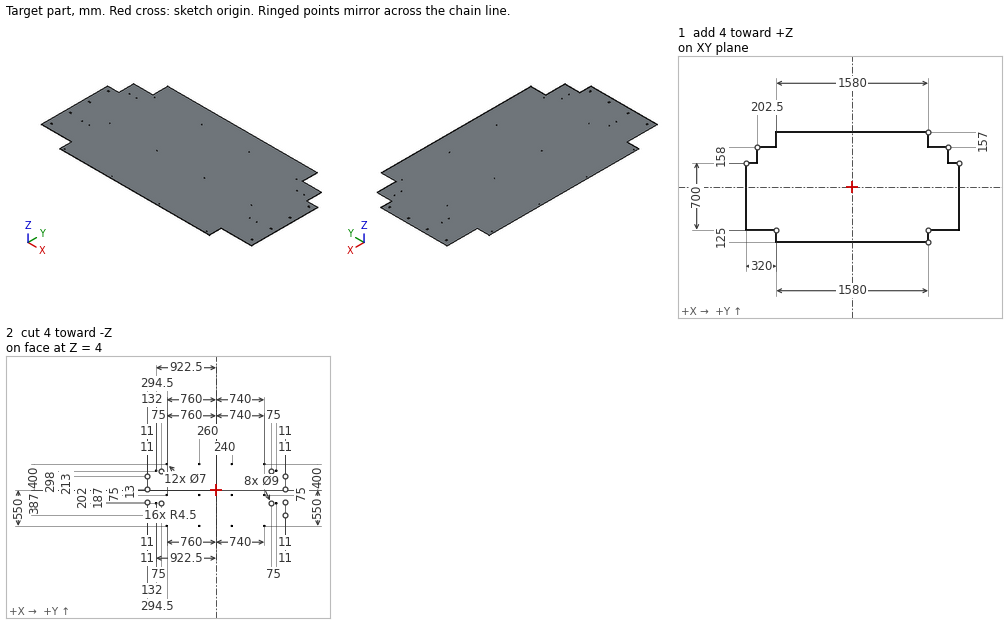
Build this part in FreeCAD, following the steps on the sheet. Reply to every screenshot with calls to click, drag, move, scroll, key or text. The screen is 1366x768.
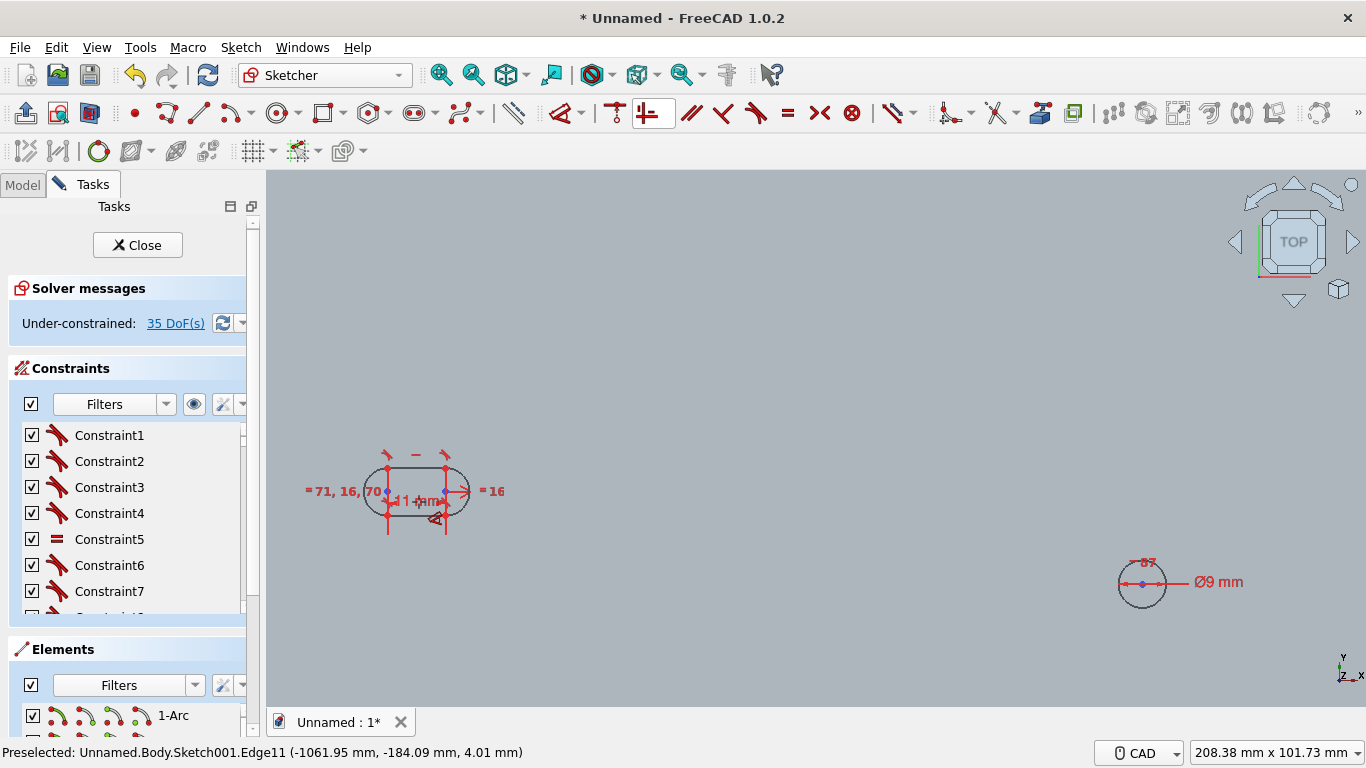
scroll(406, 474, down, 14)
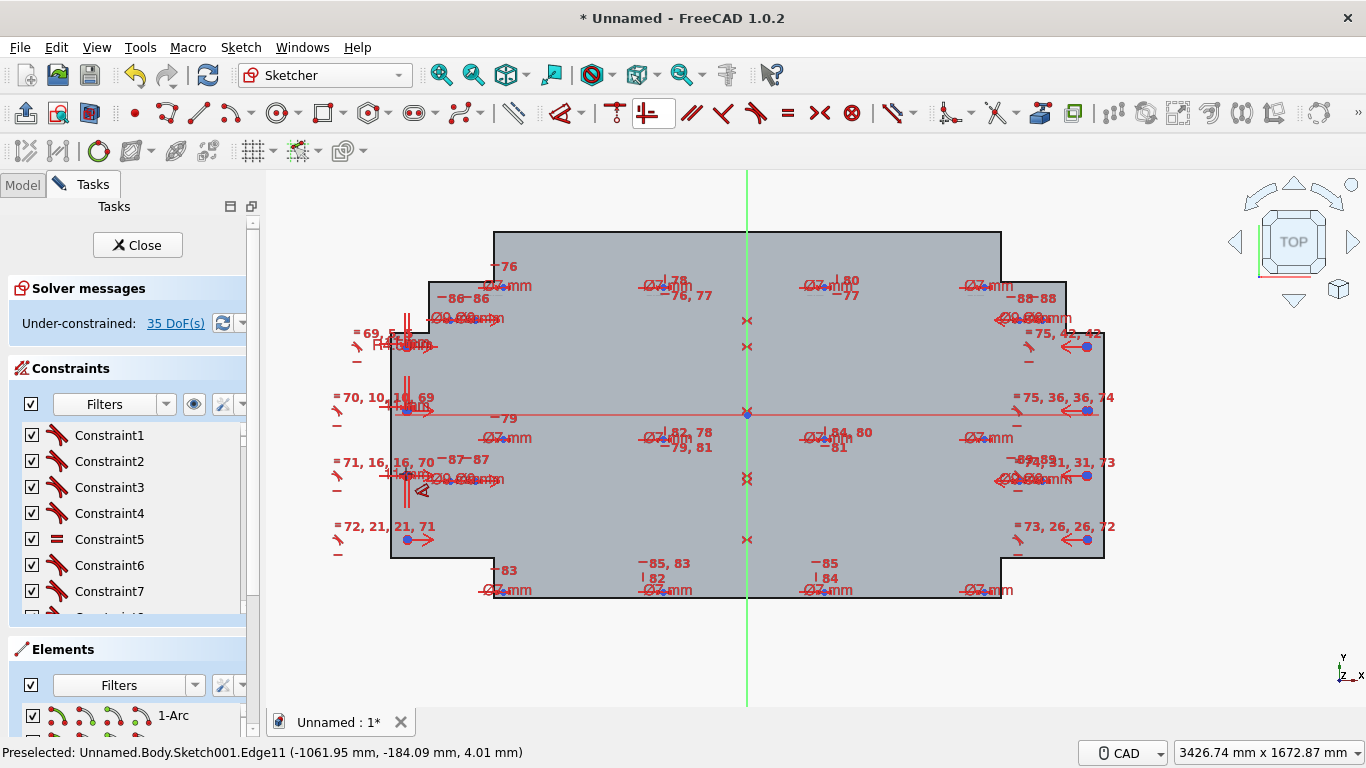
scroll(407, 538, up, 14)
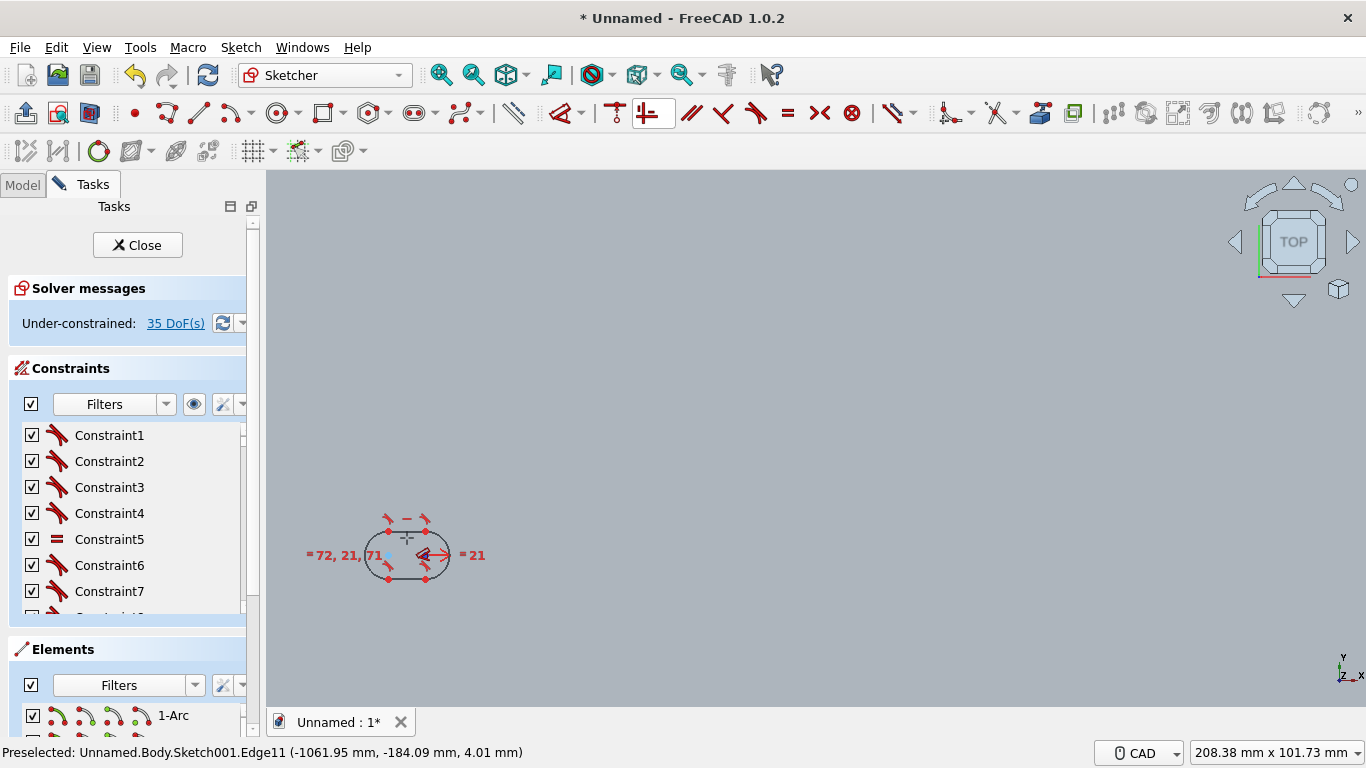
click(400, 532)
click(407, 566)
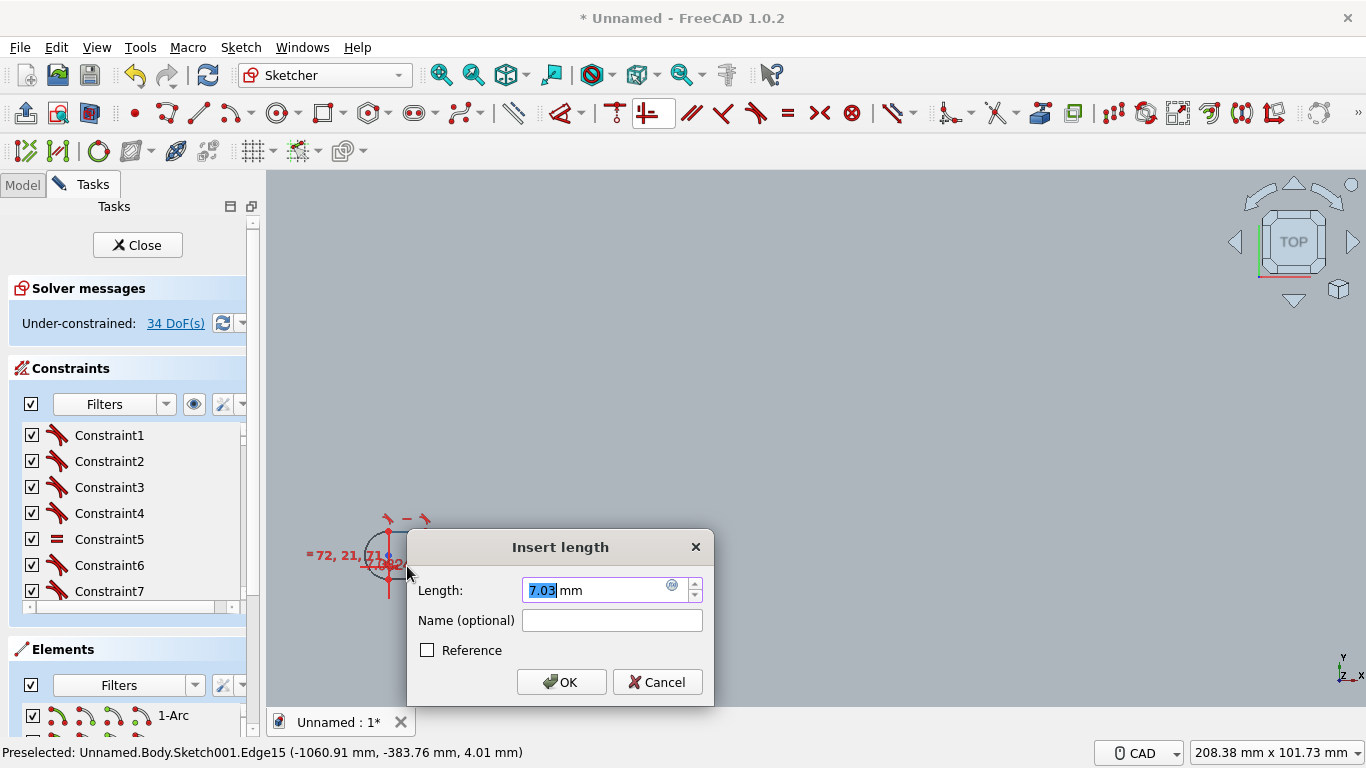
text(11)
key(Return)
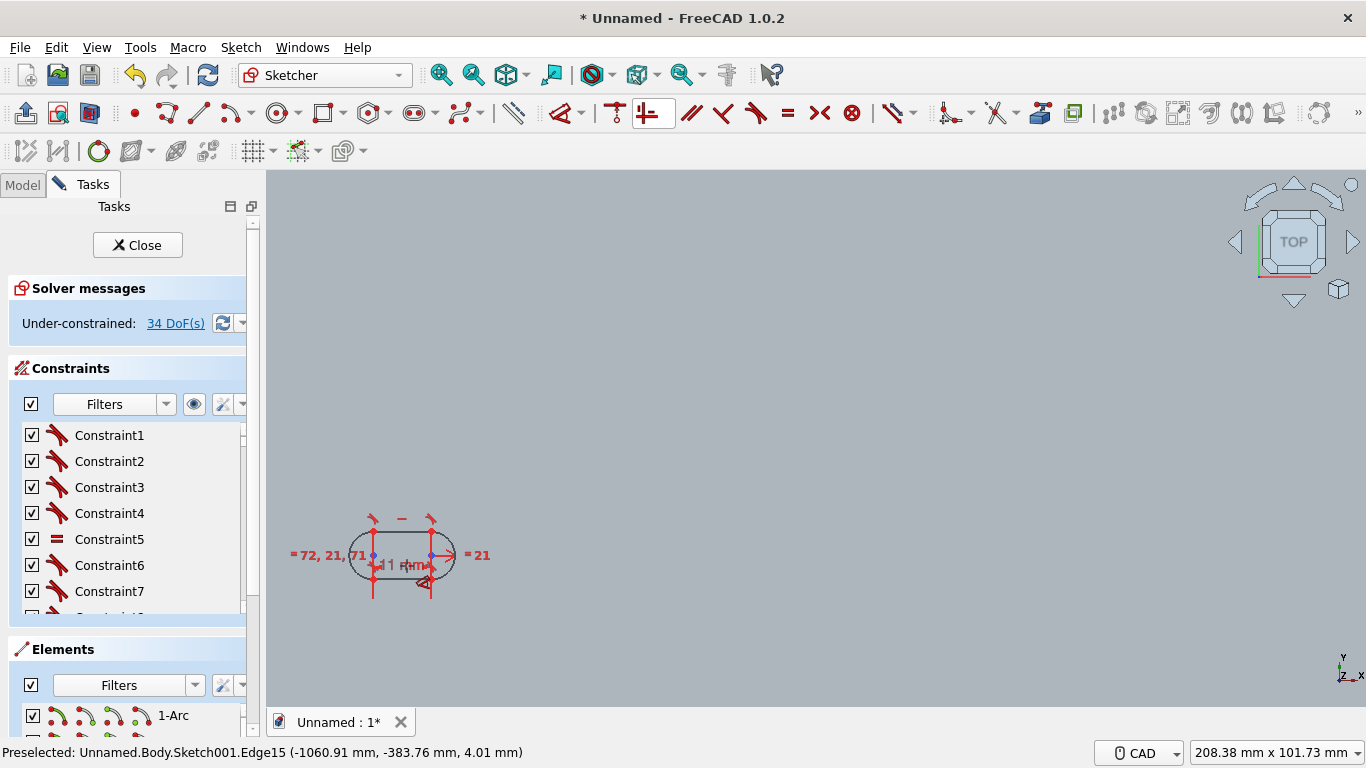
scroll(407, 538, down, 14)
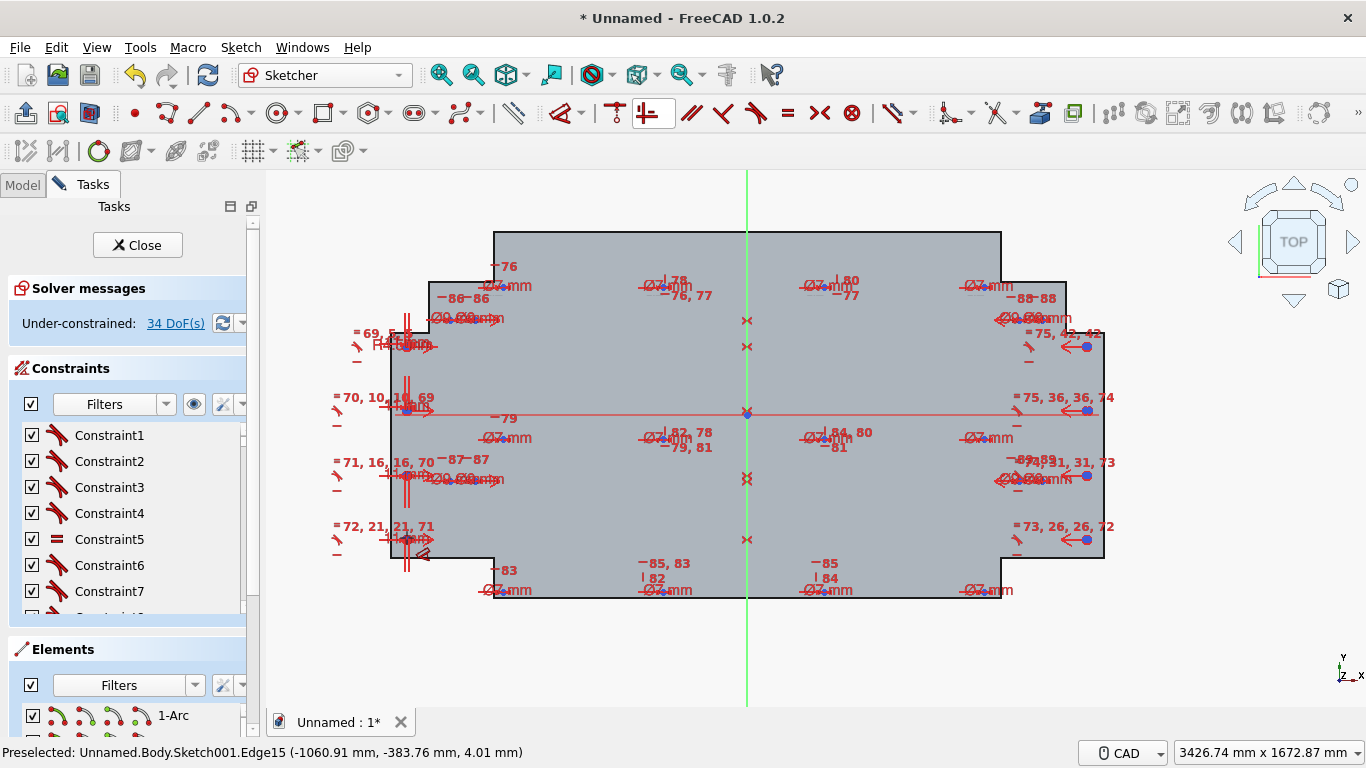
scroll(1087, 538, up, 14)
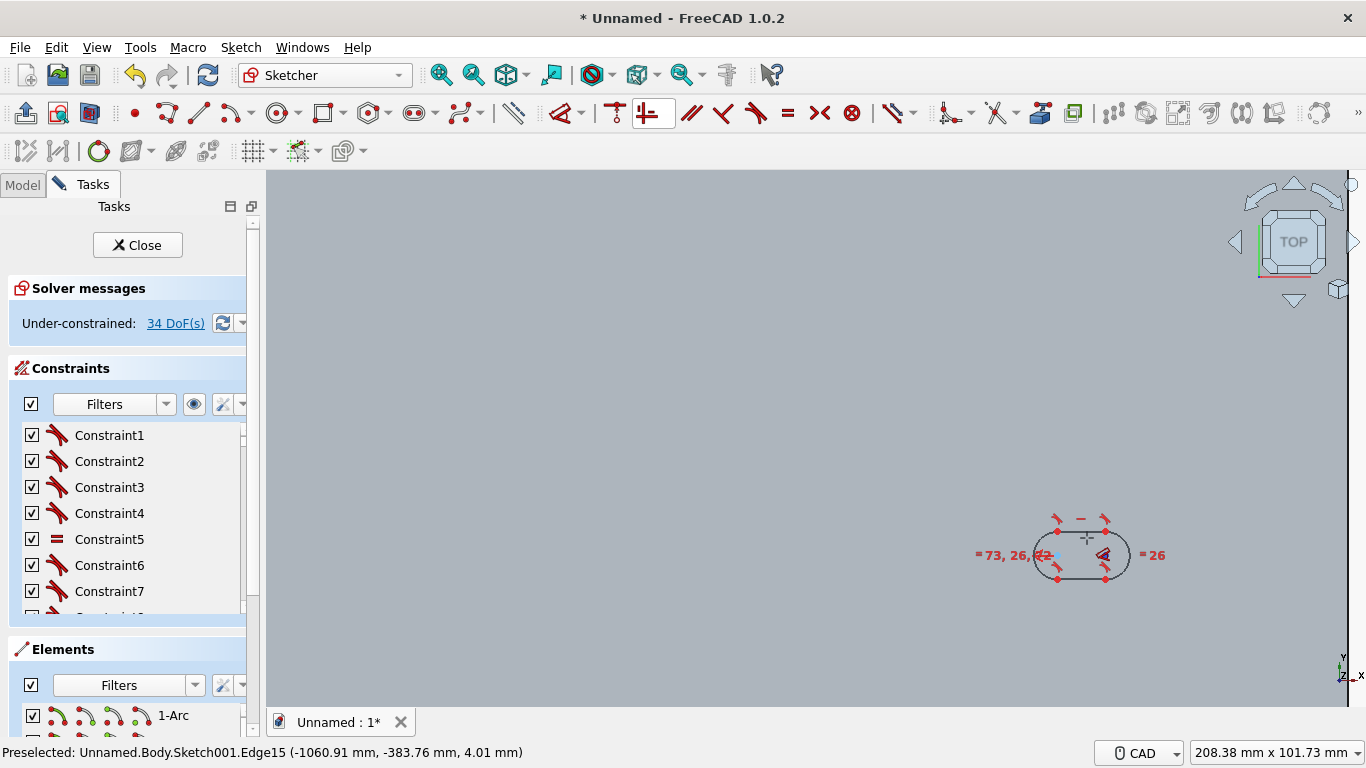
click(1072, 532)
click(1082, 566)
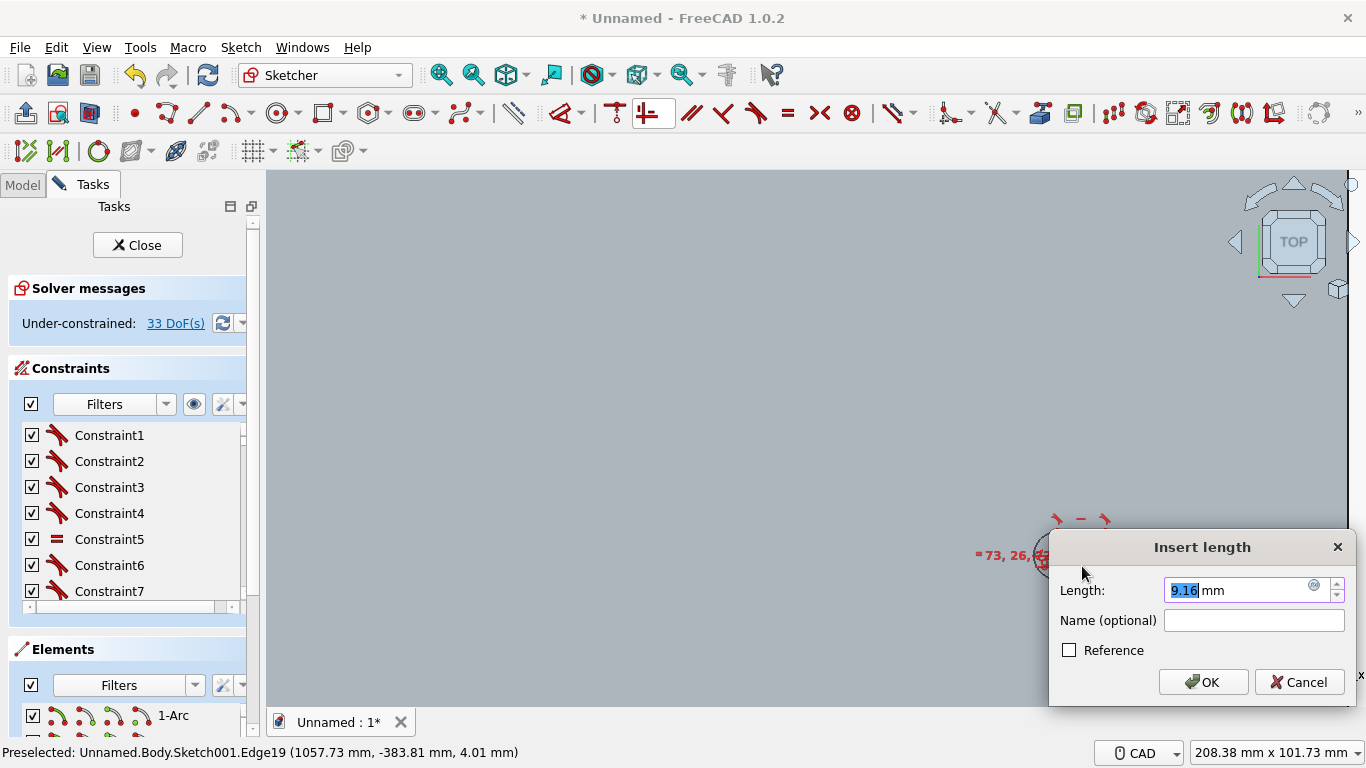
text(11)
key(Return)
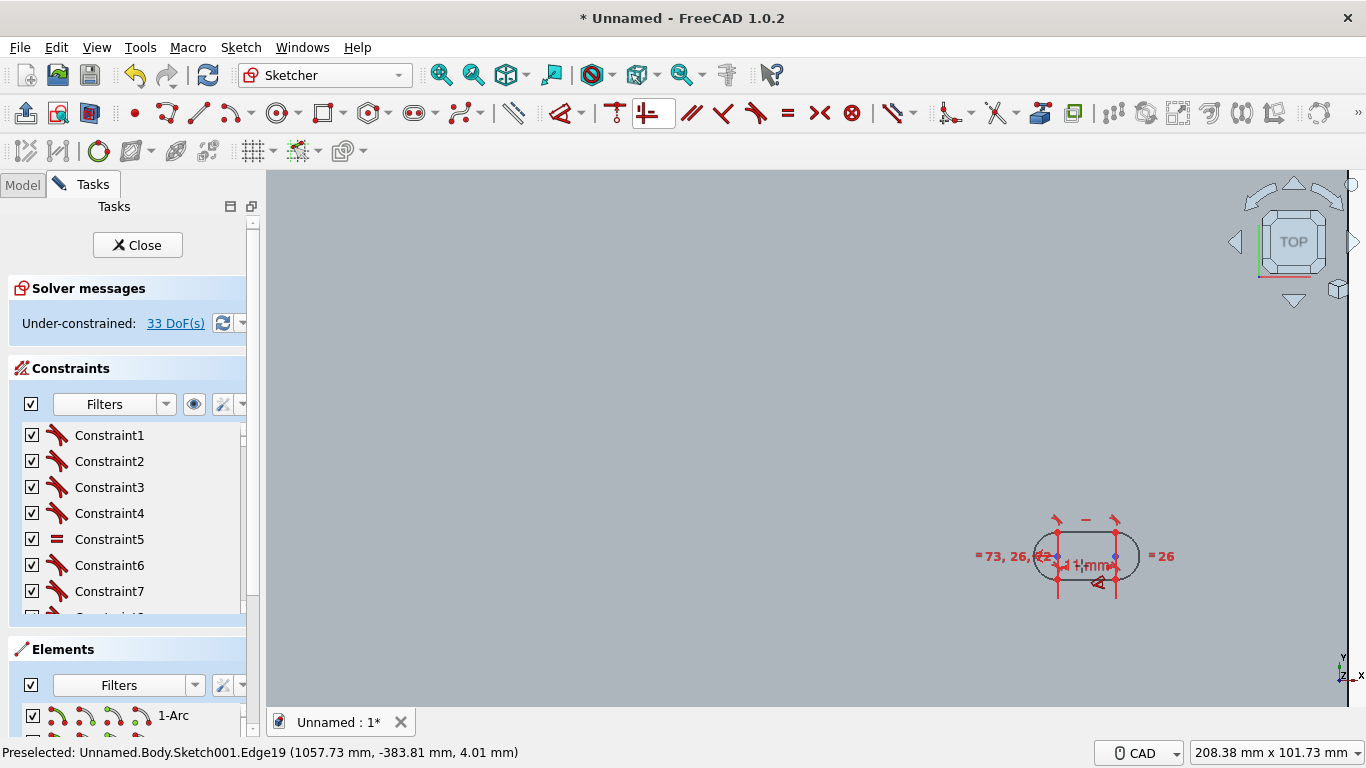
scroll(1088, 538, down, 14)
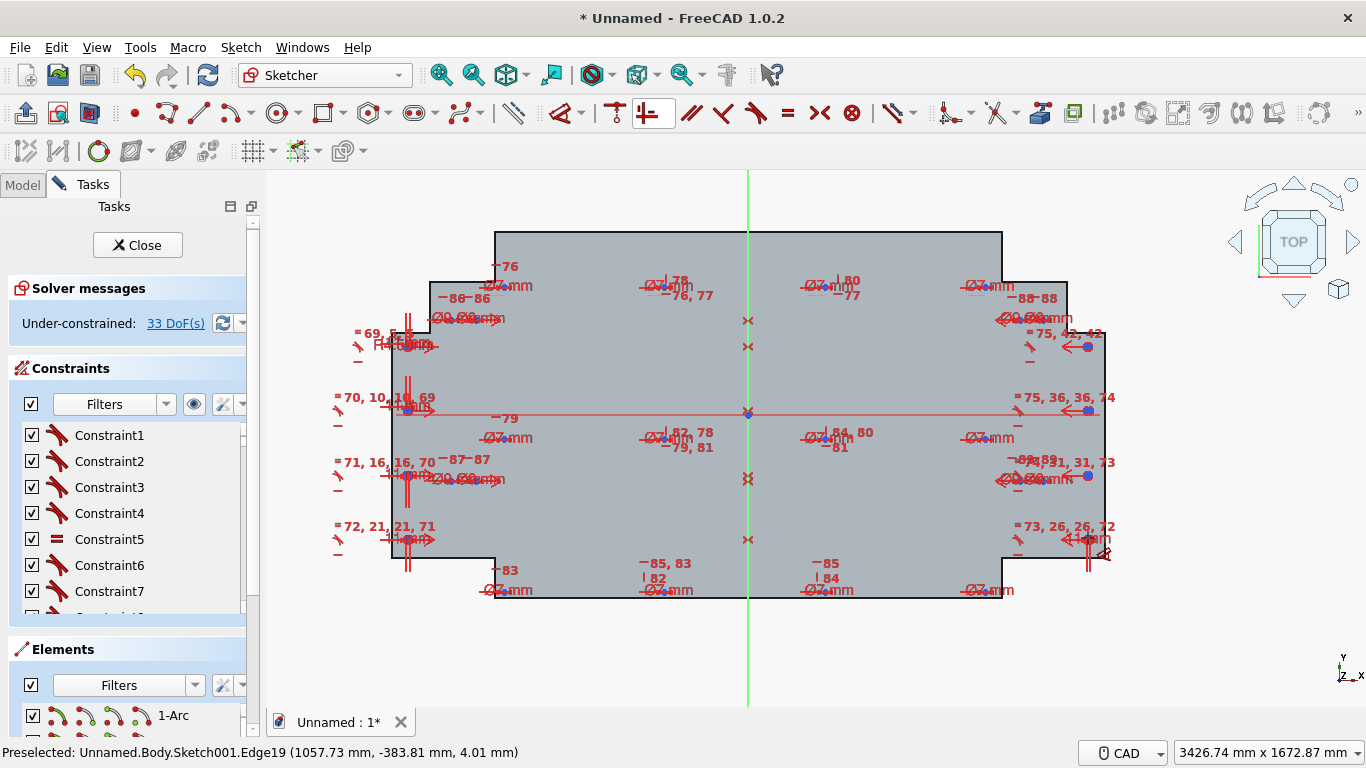
scroll(1088, 474, up, 14)